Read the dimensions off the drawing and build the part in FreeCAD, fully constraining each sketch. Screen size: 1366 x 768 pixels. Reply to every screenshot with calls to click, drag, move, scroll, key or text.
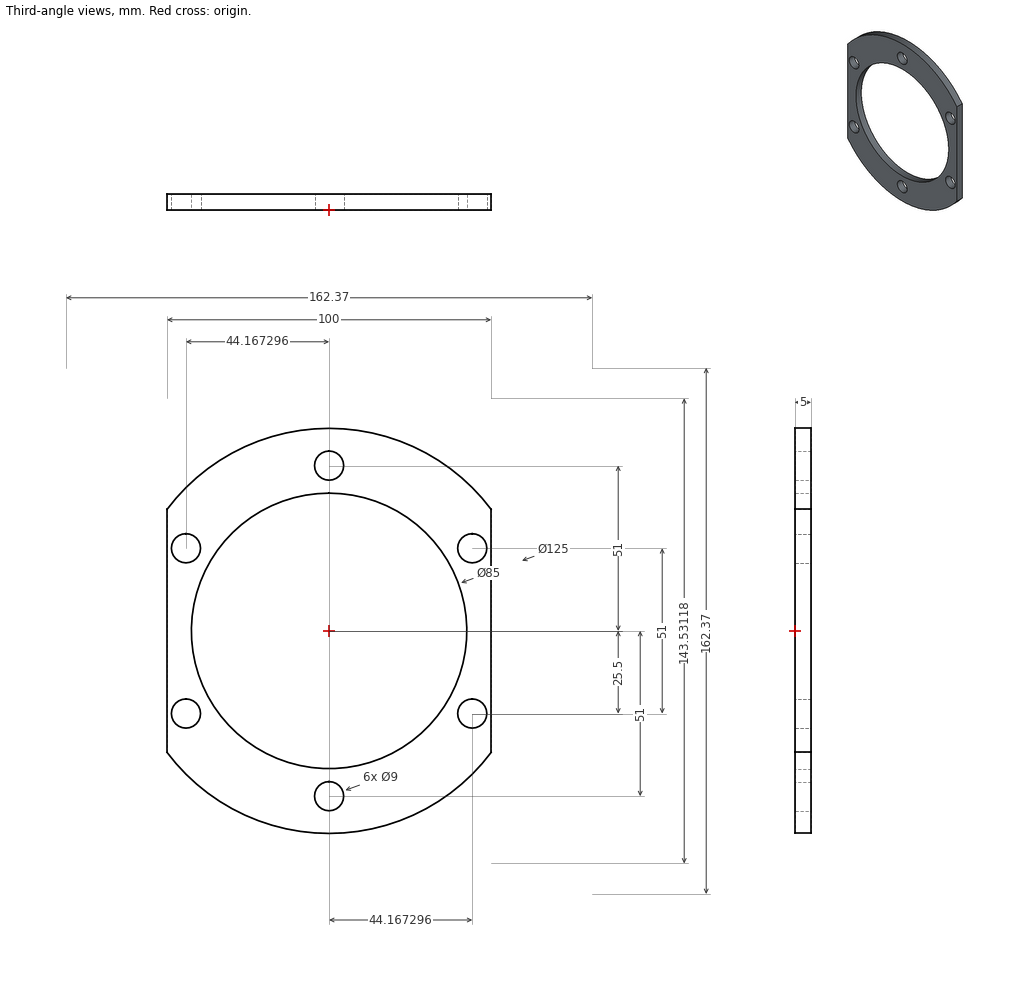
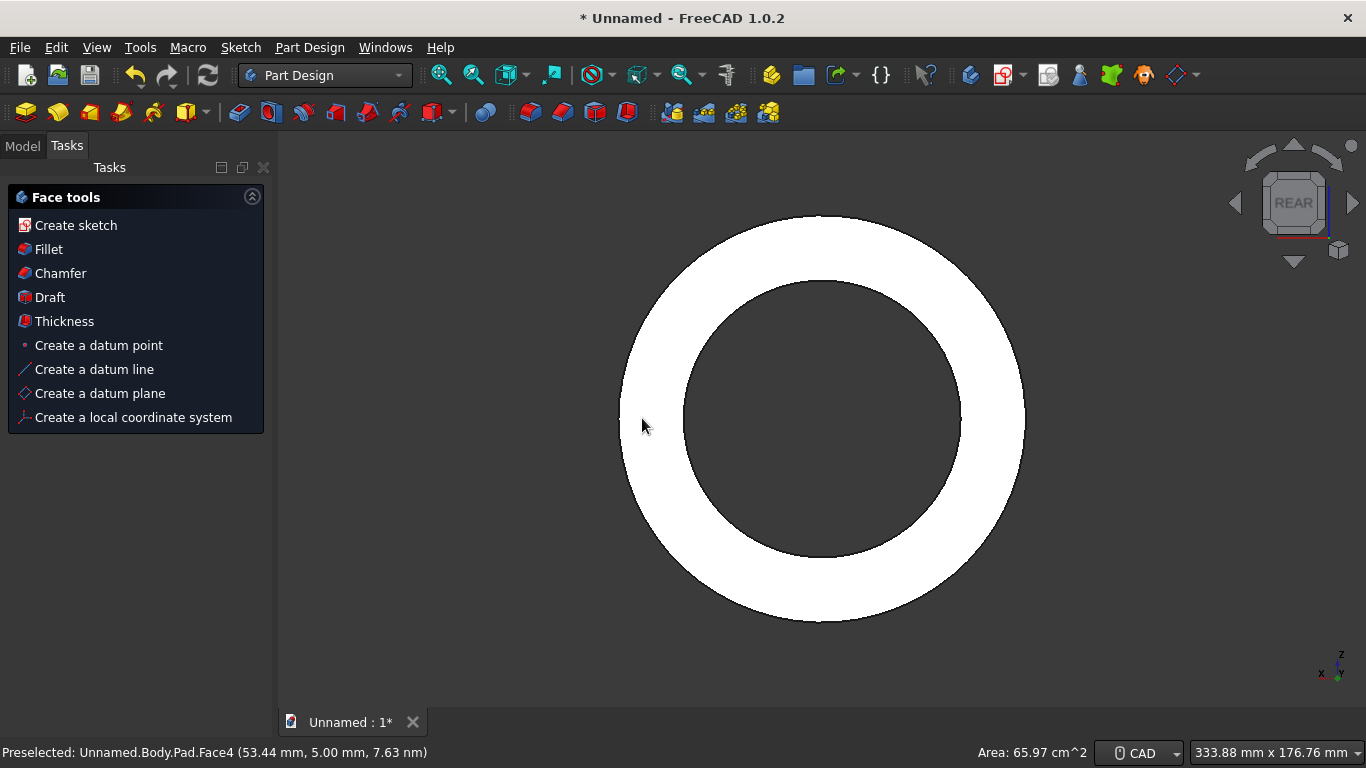
click(1004, 76)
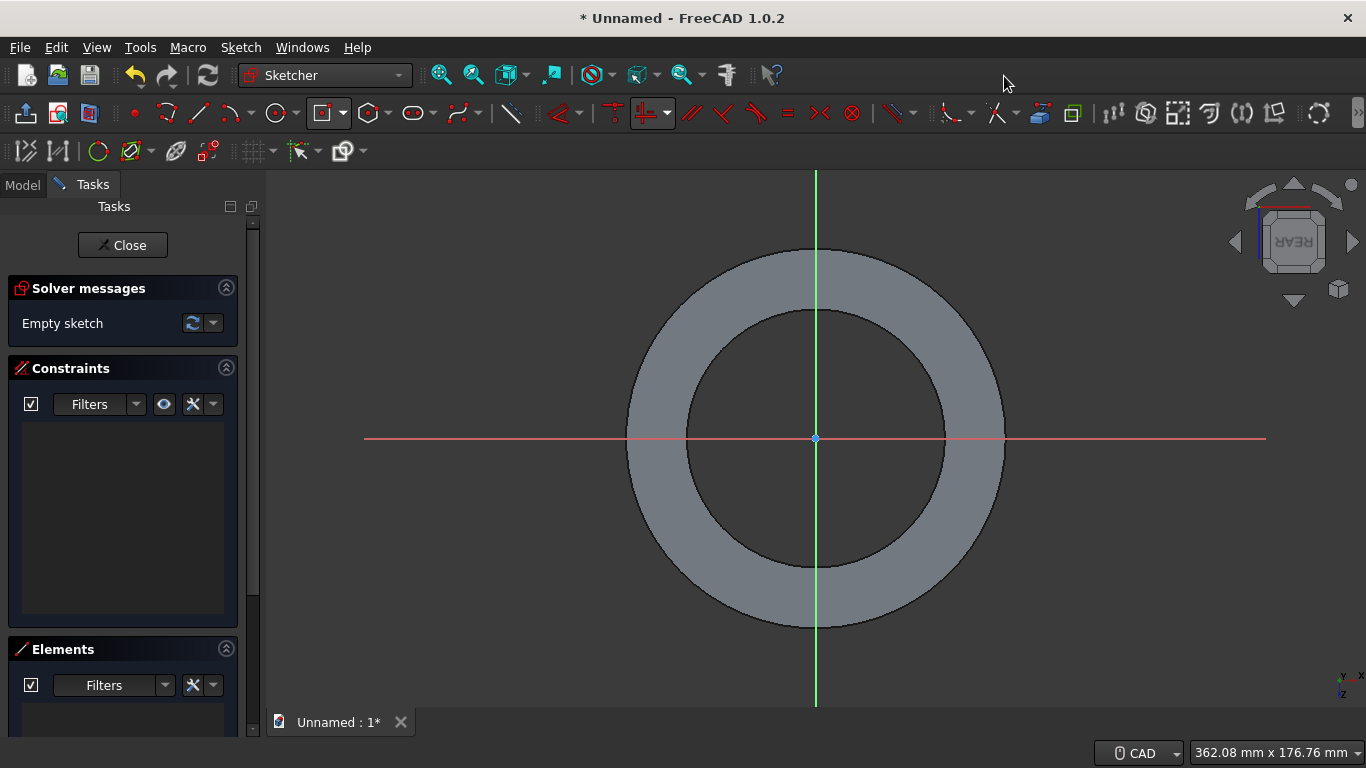
click(276, 114)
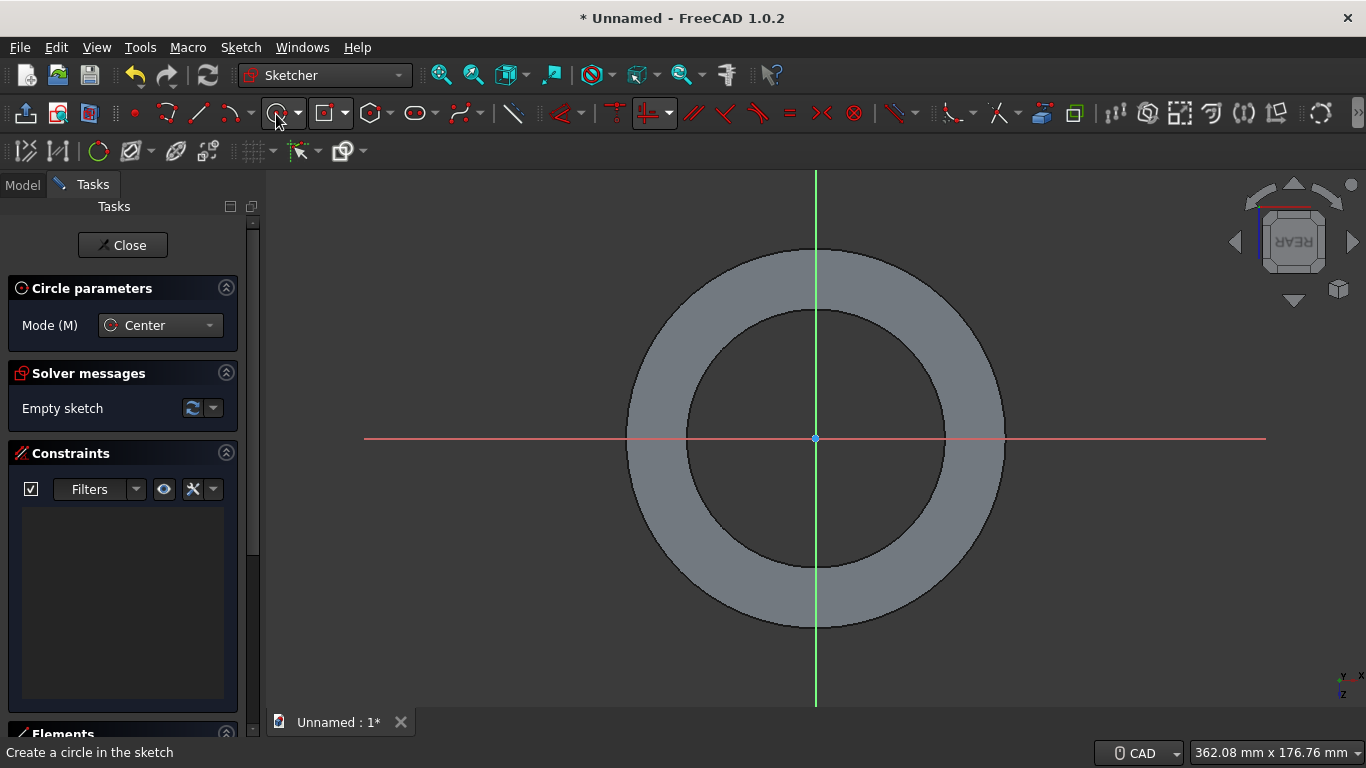
scroll(816, 284, up, 3)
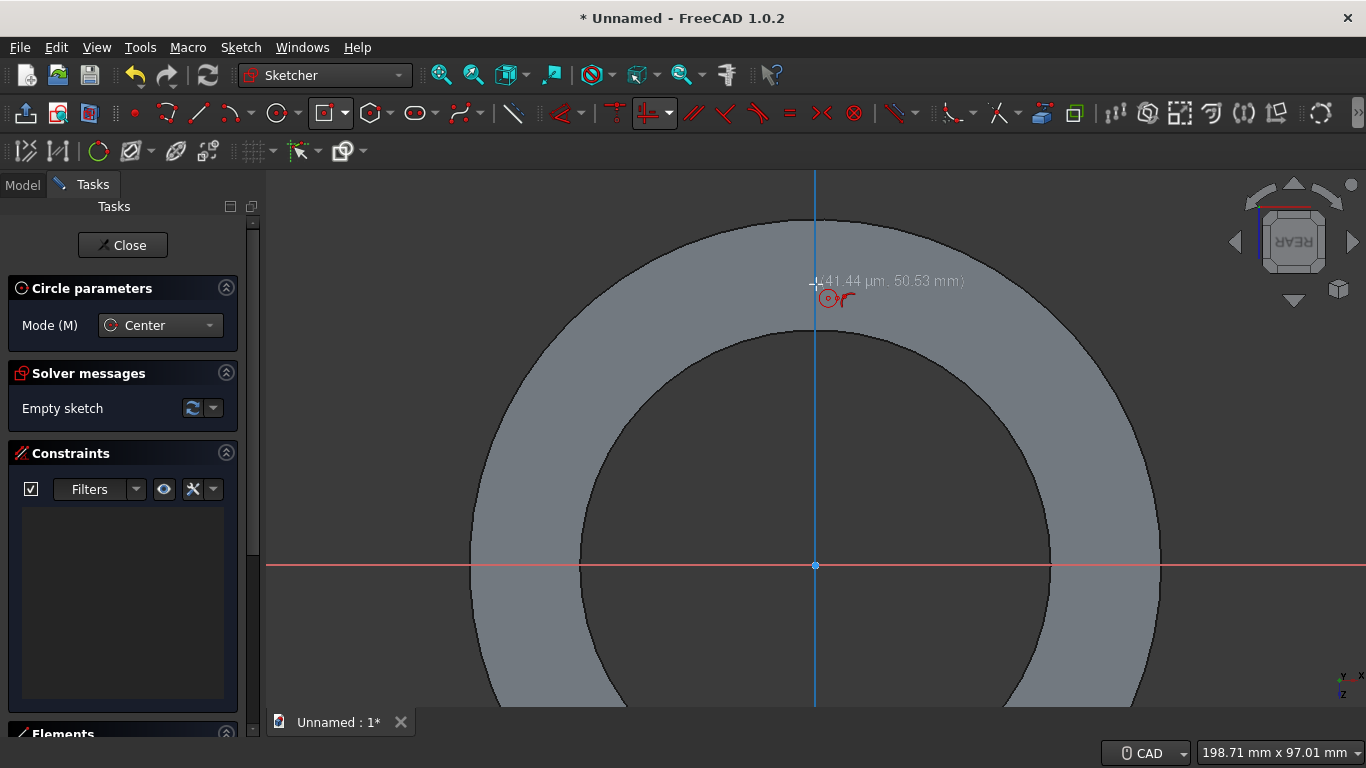
click(815, 283)
move(833, 265)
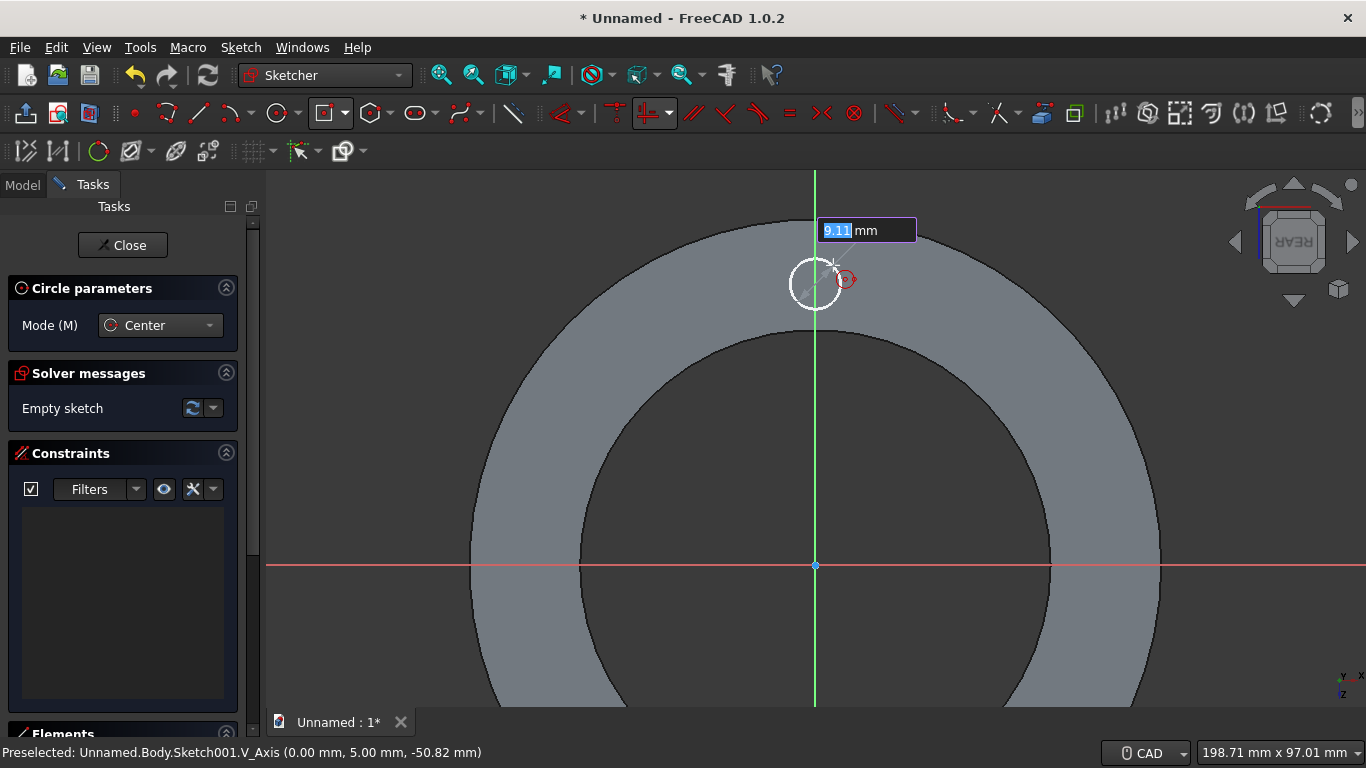
text(9)
key(Return)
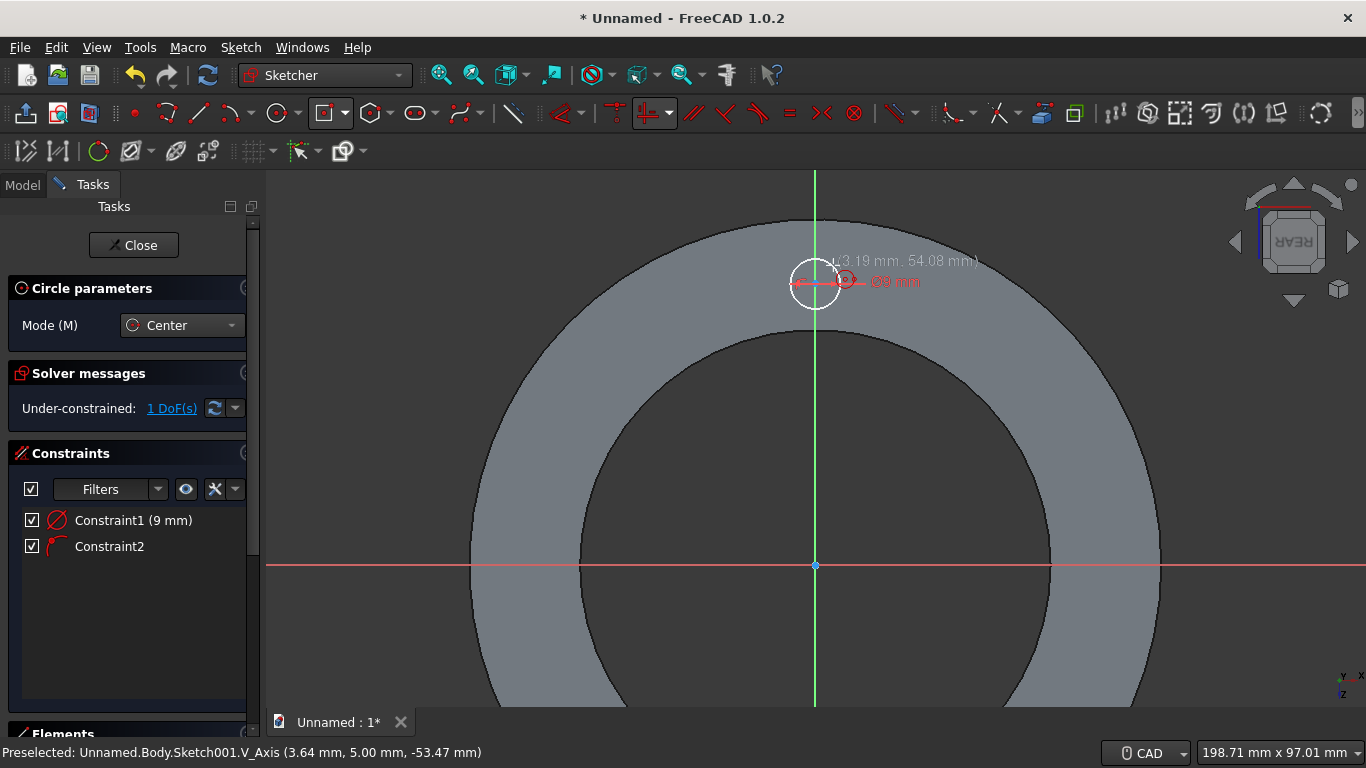
click(1060, 424)
move(1077, 407)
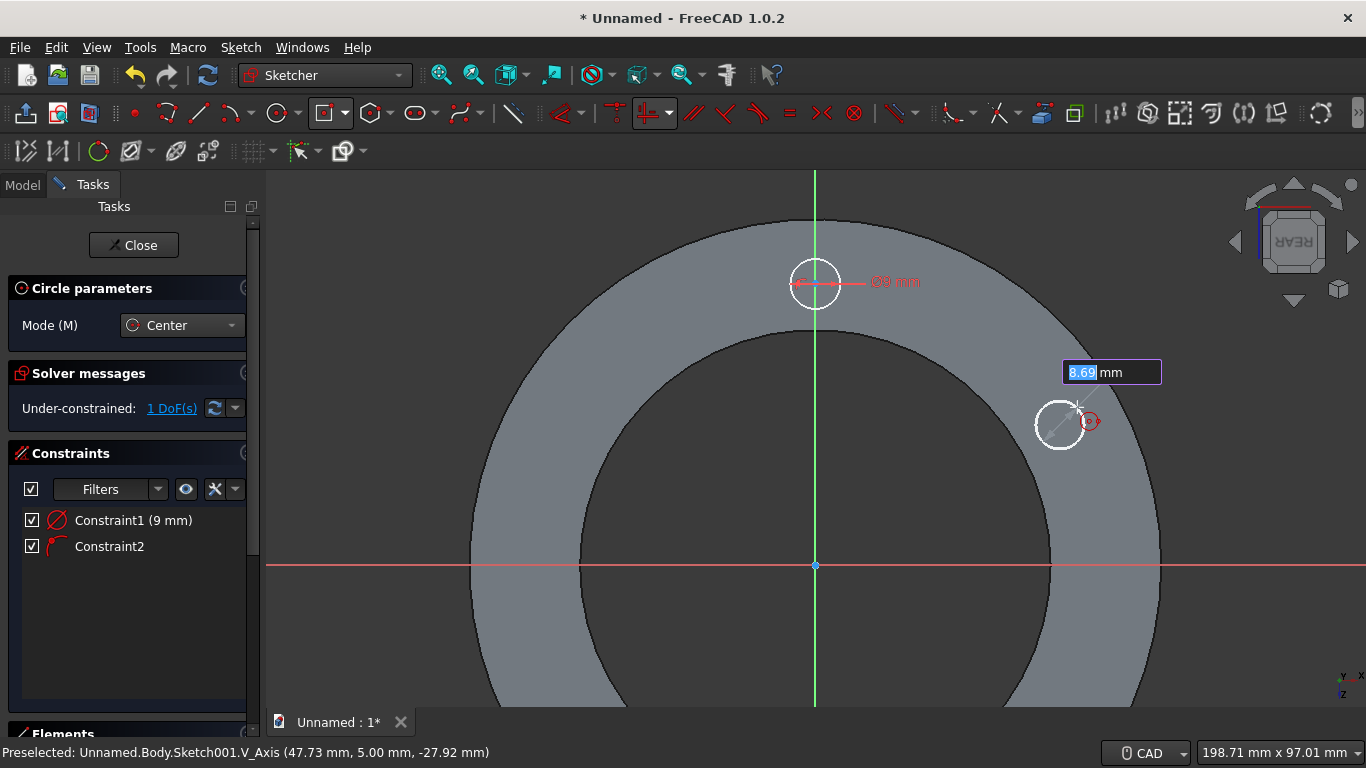
text(9)
key(Return)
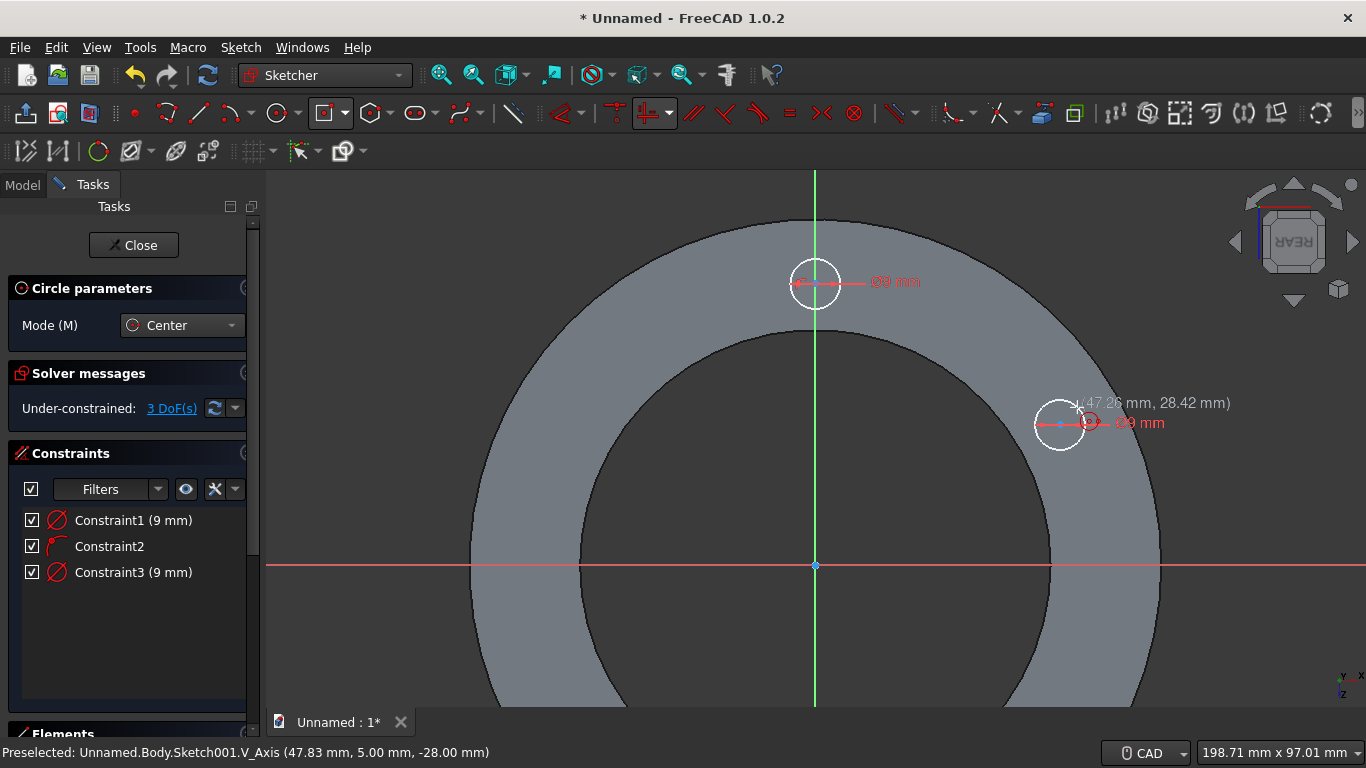
scroll(665, 284, down, 3)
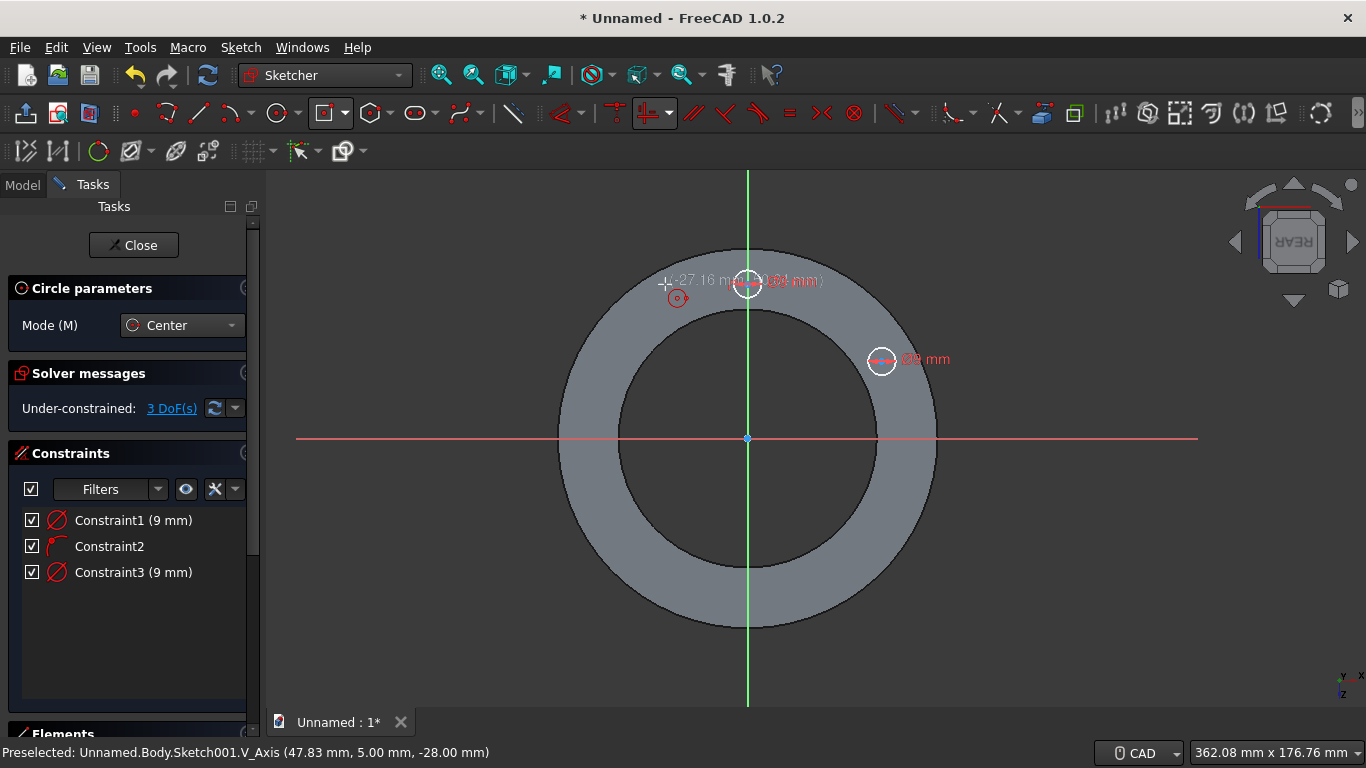
scroll(882, 516, up, 3)